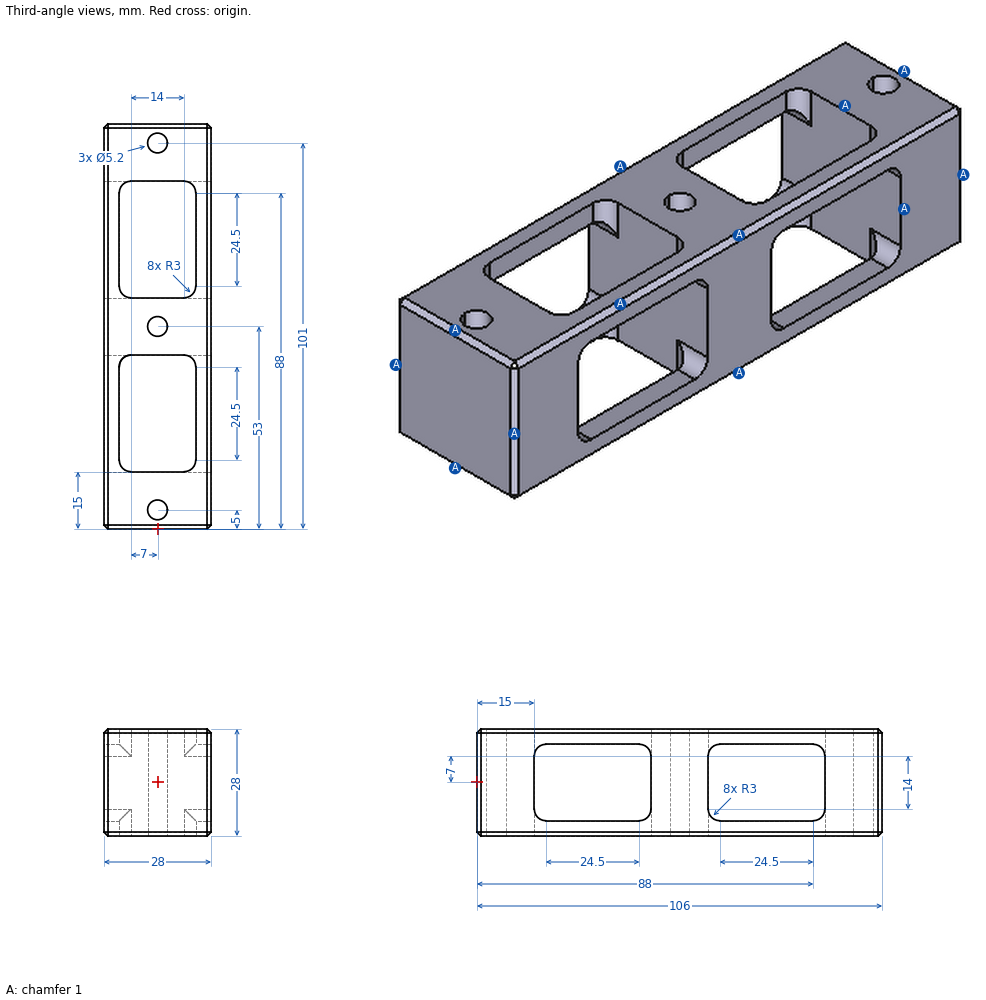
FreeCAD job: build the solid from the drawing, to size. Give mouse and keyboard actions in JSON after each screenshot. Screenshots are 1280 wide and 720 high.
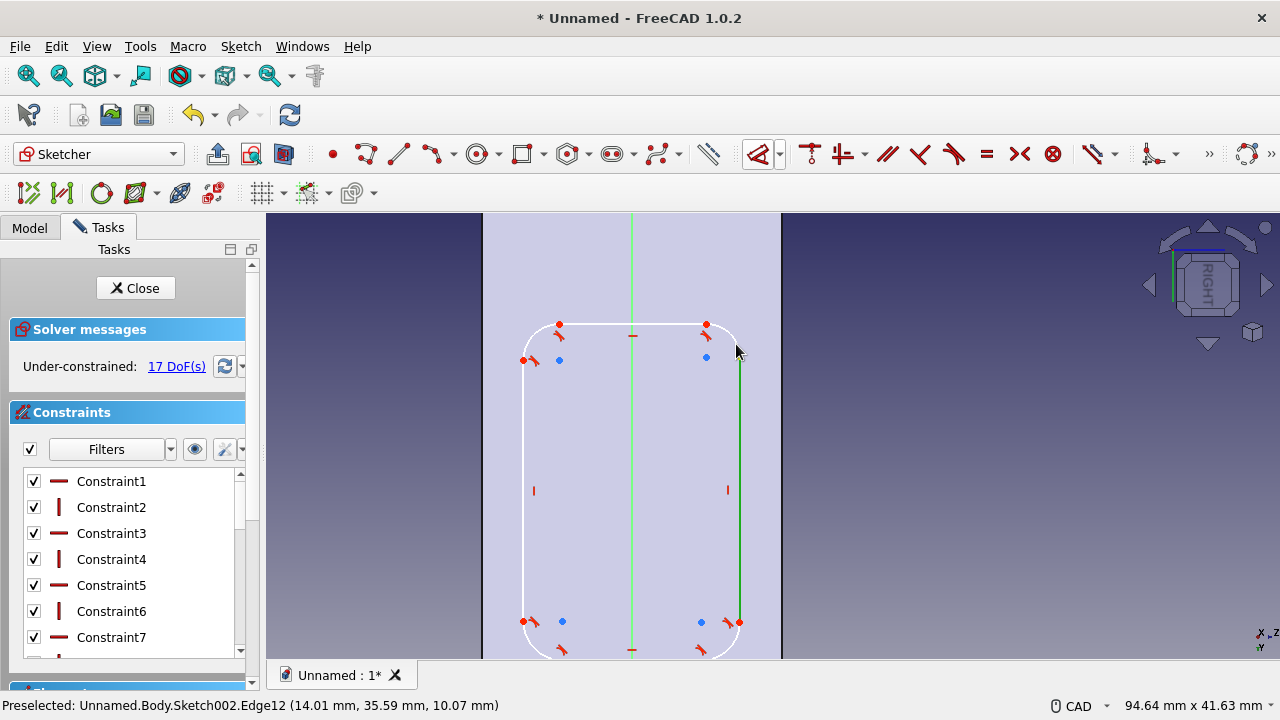
{"action": "left_click", "coordinate": [736, 342]}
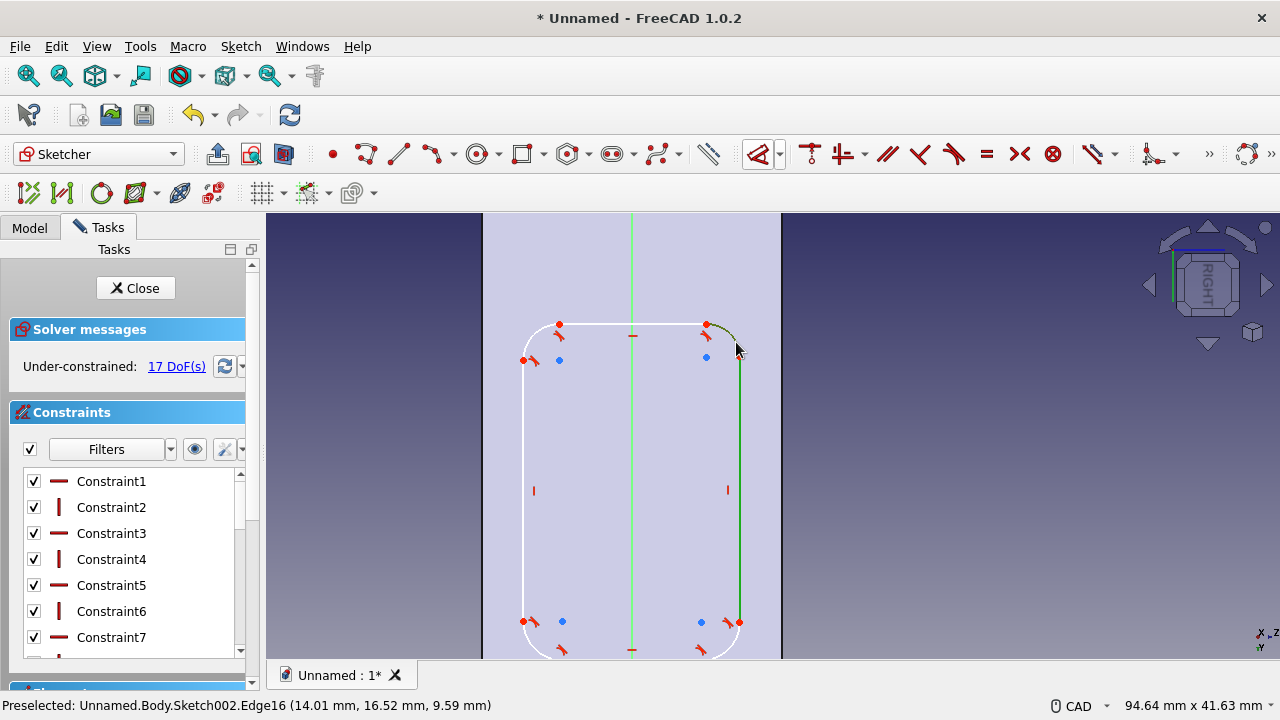
{"action": "left_click", "coordinate": [954, 154]}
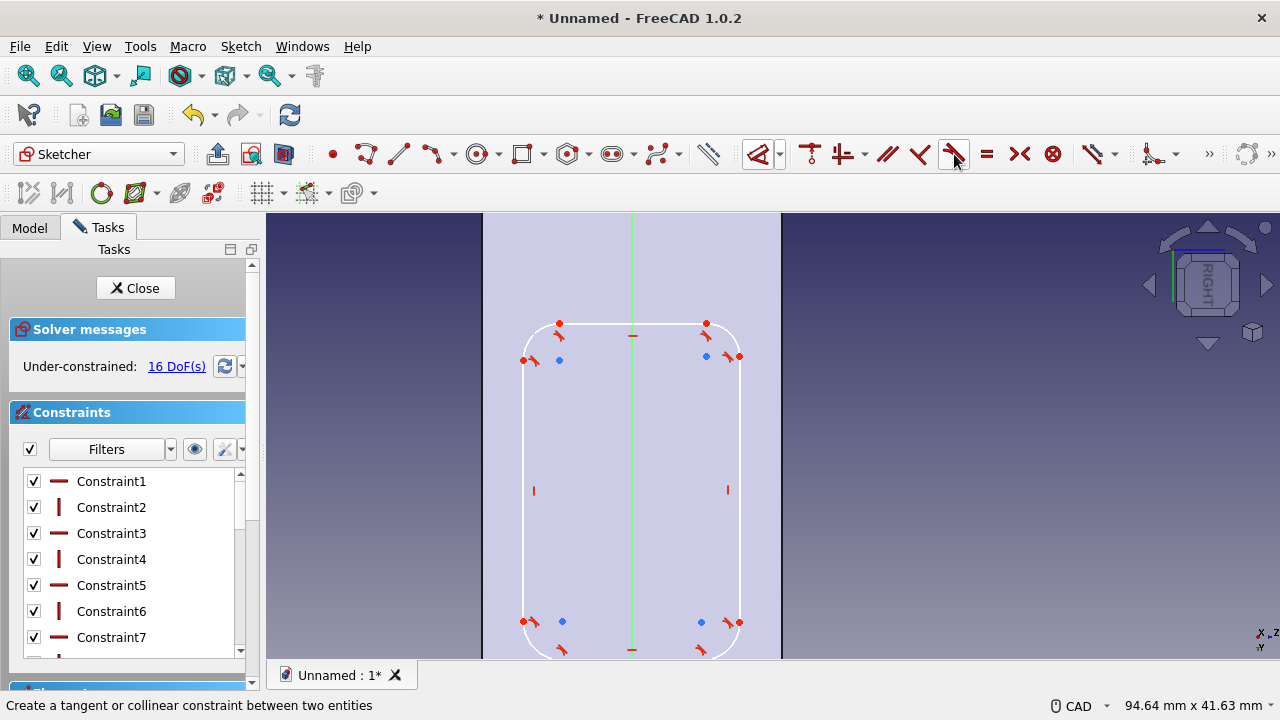
{"action": "scroll", "coordinate": [736, 344], "scroll_direction": "down", "scroll_amount": 6}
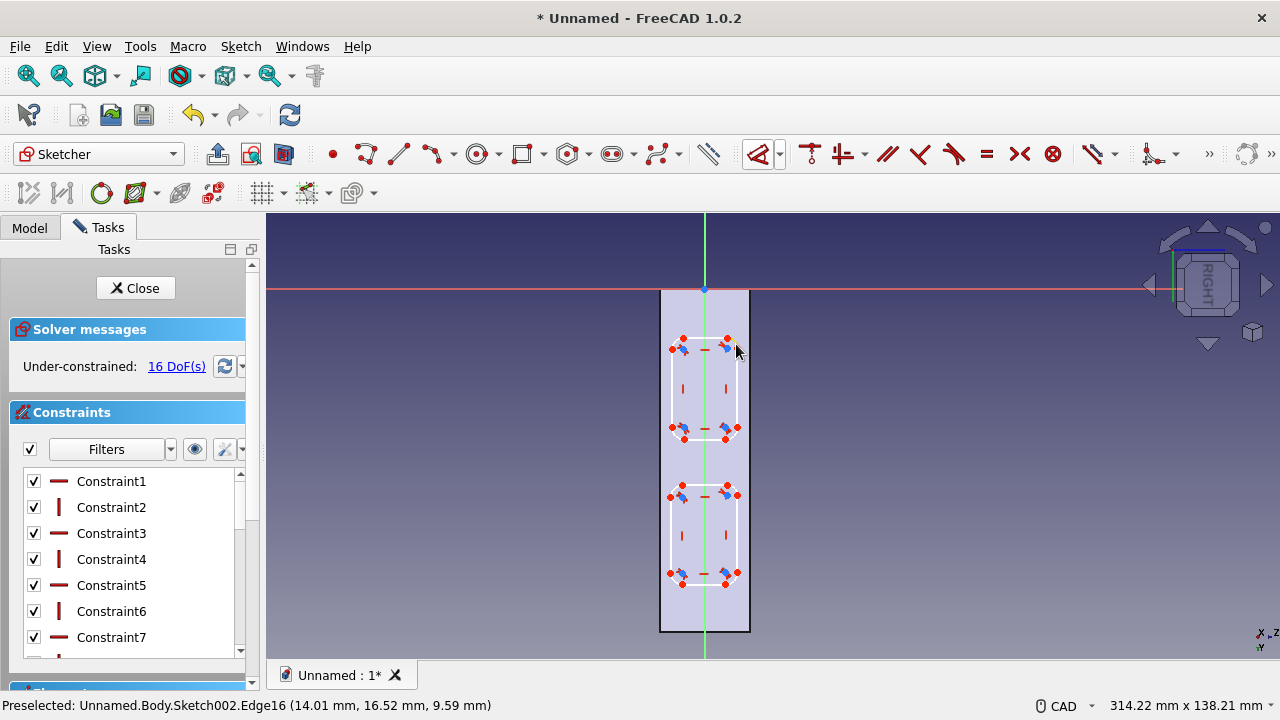
{"action": "scroll", "coordinate": [677, 487], "scroll_direction": "up", "scroll_amount": 5}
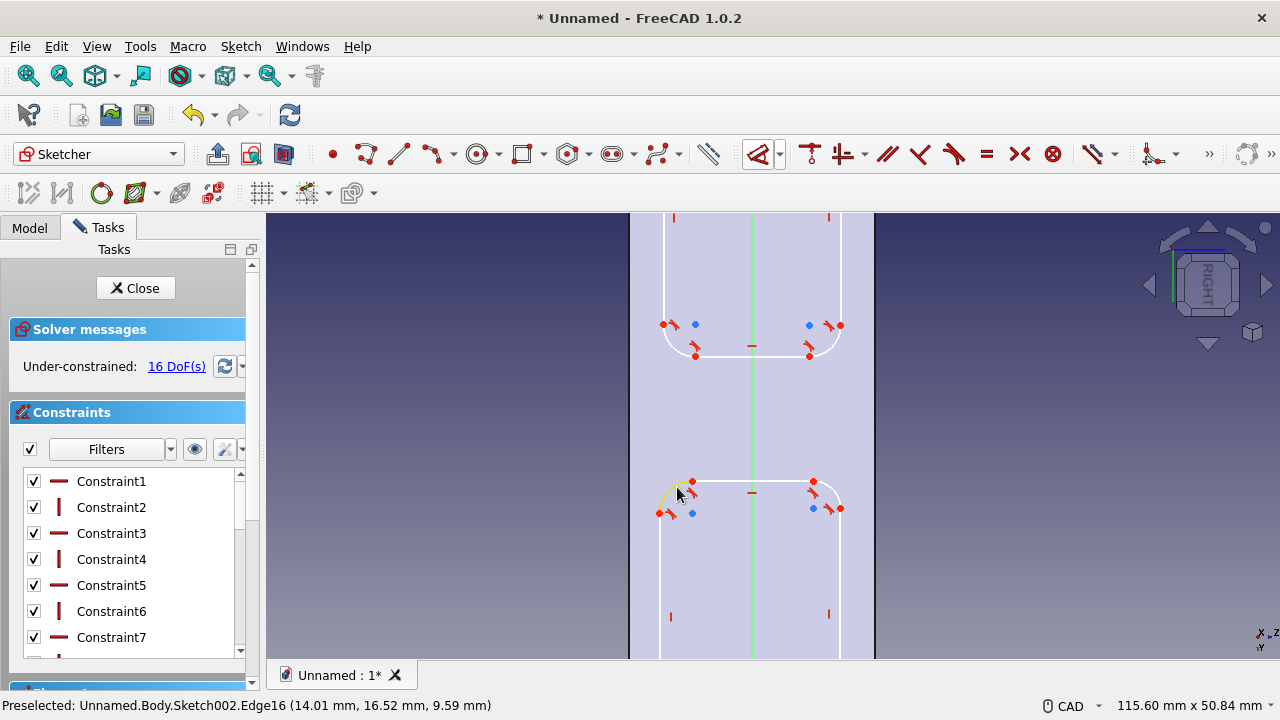
{"action": "left_click", "coordinate": [678, 485]}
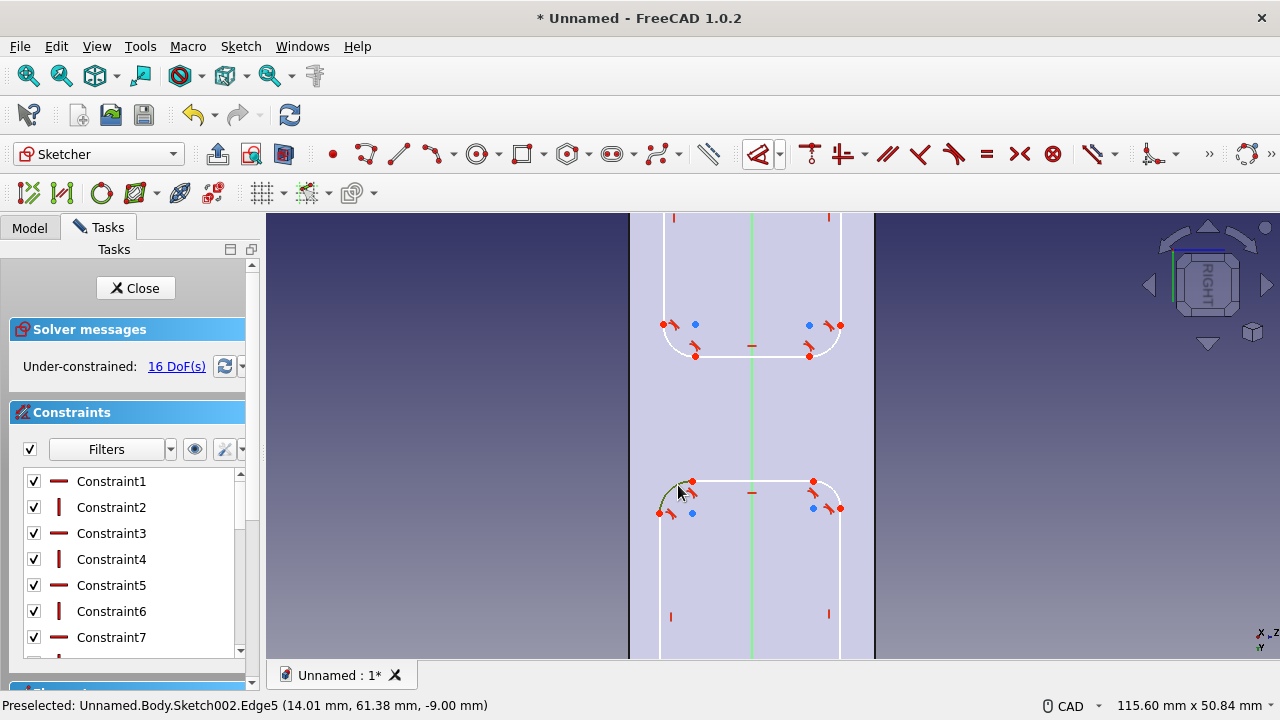
{"action": "scroll", "coordinate": [677, 487], "scroll_direction": "down", "scroll_amount": 5}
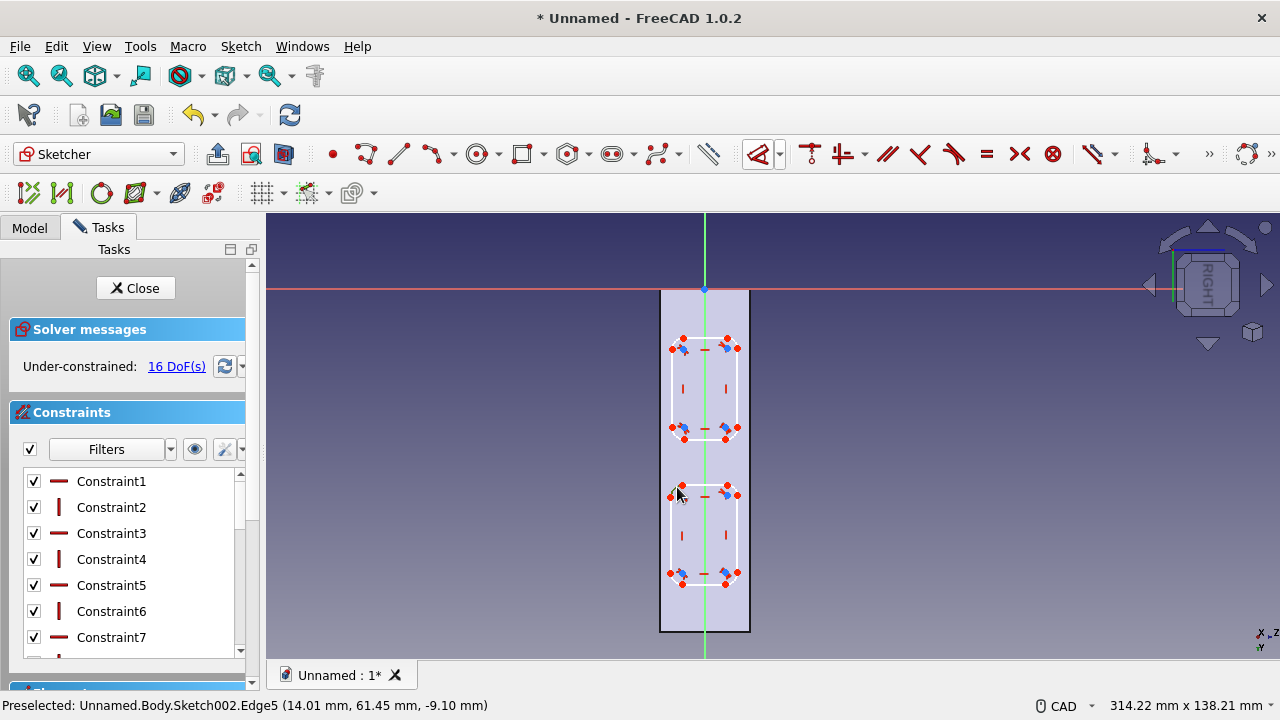
{"action": "scroll", "coordinate": [672, 578], "scroll_direction": "up", "scroll_amount": 5}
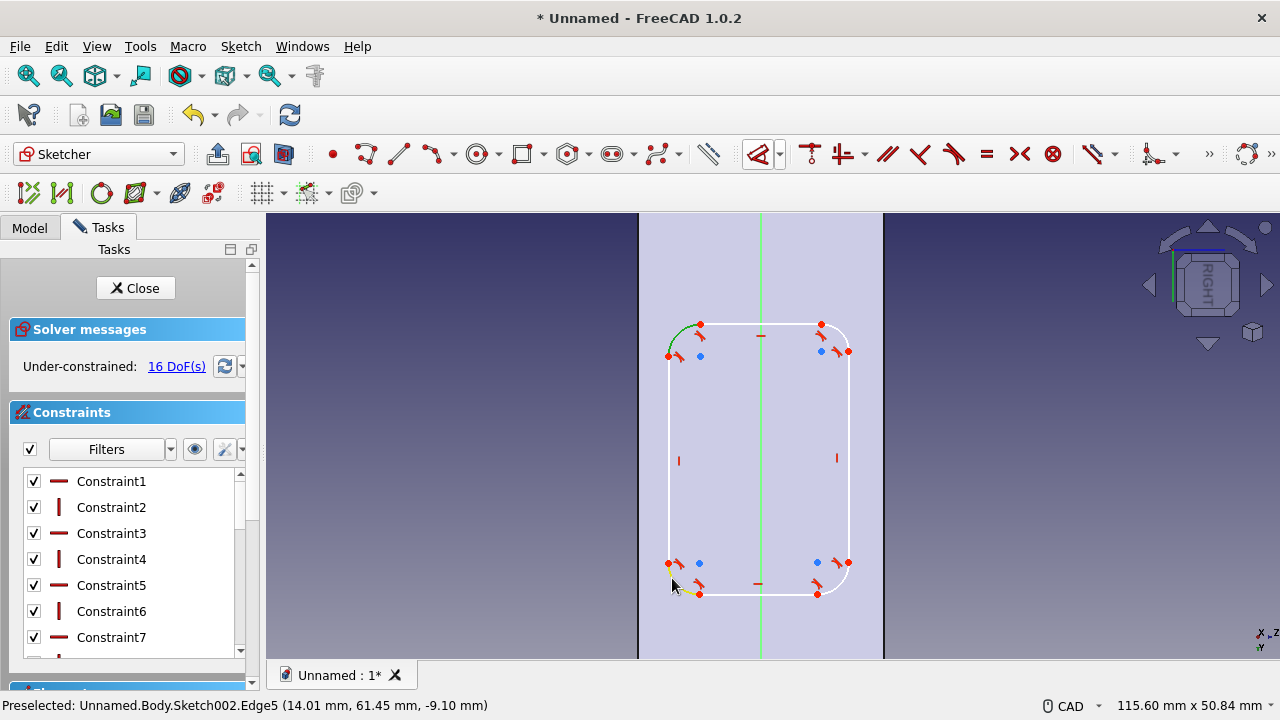
{"action": "left_click", "coordinate": [672, 577]}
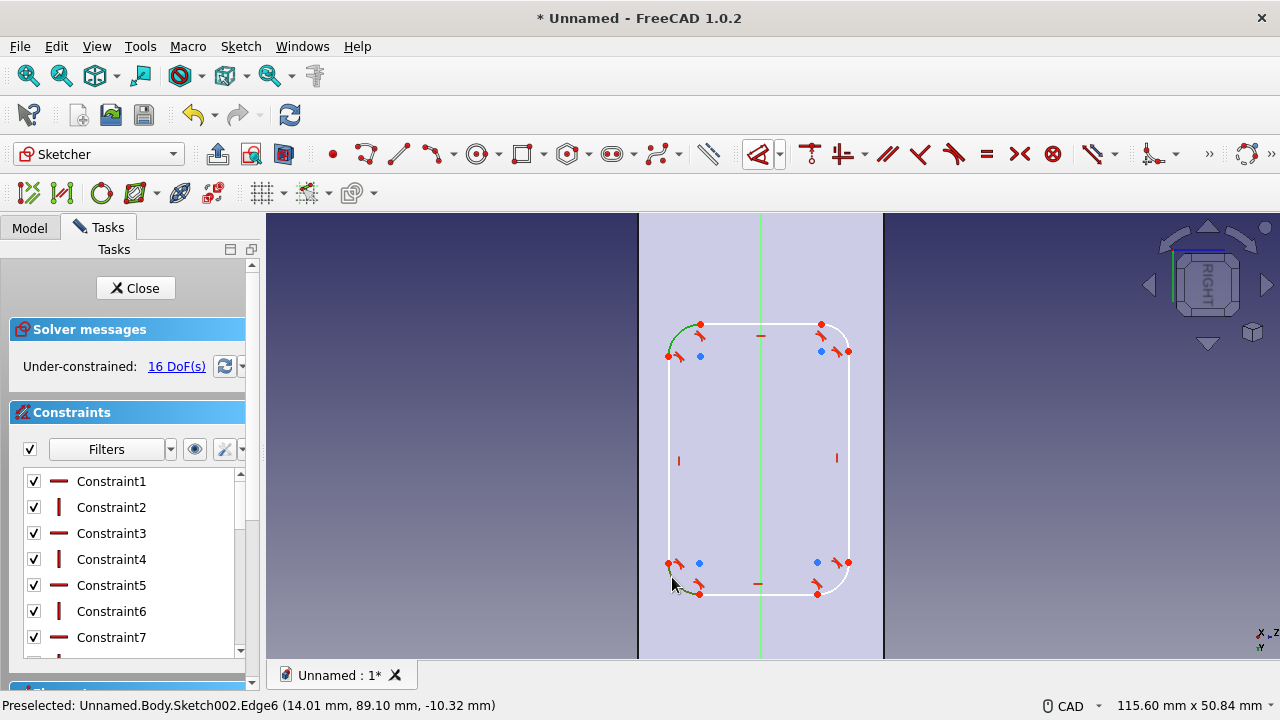
{"action": "left_click", "coordinate": [832, 591]}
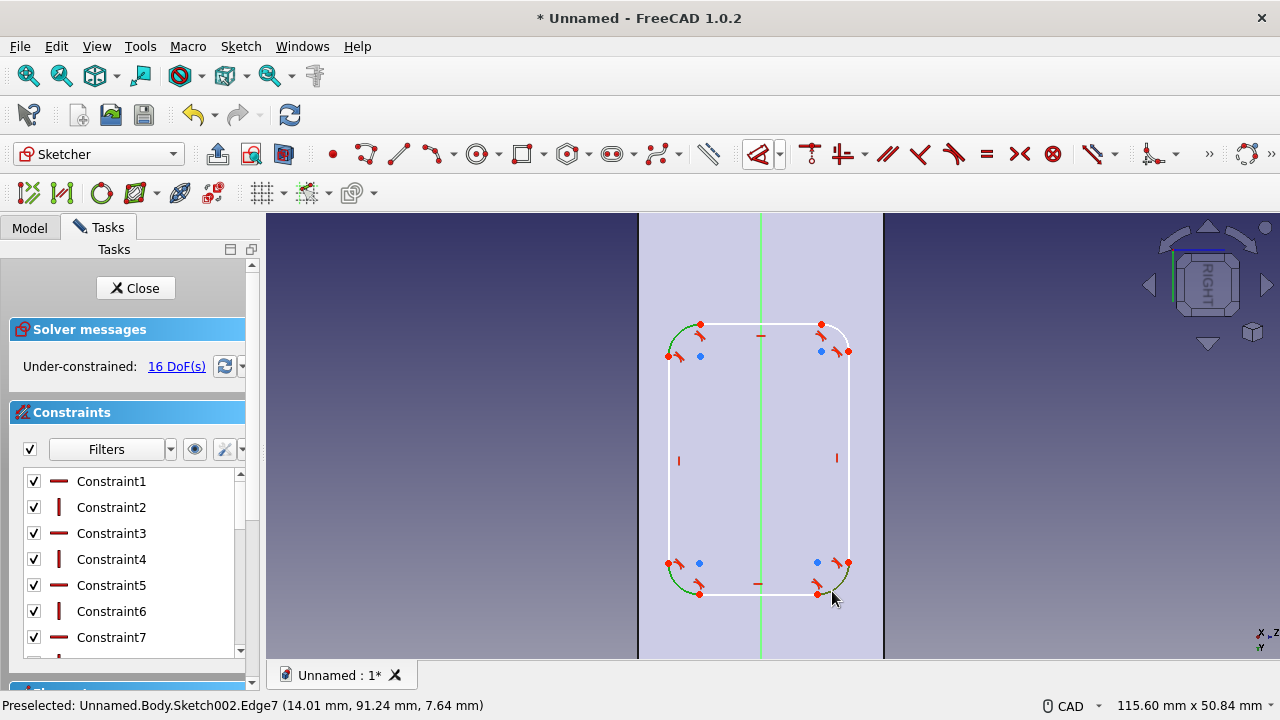
{"action": "left_click", "coordinate": [846, 339]}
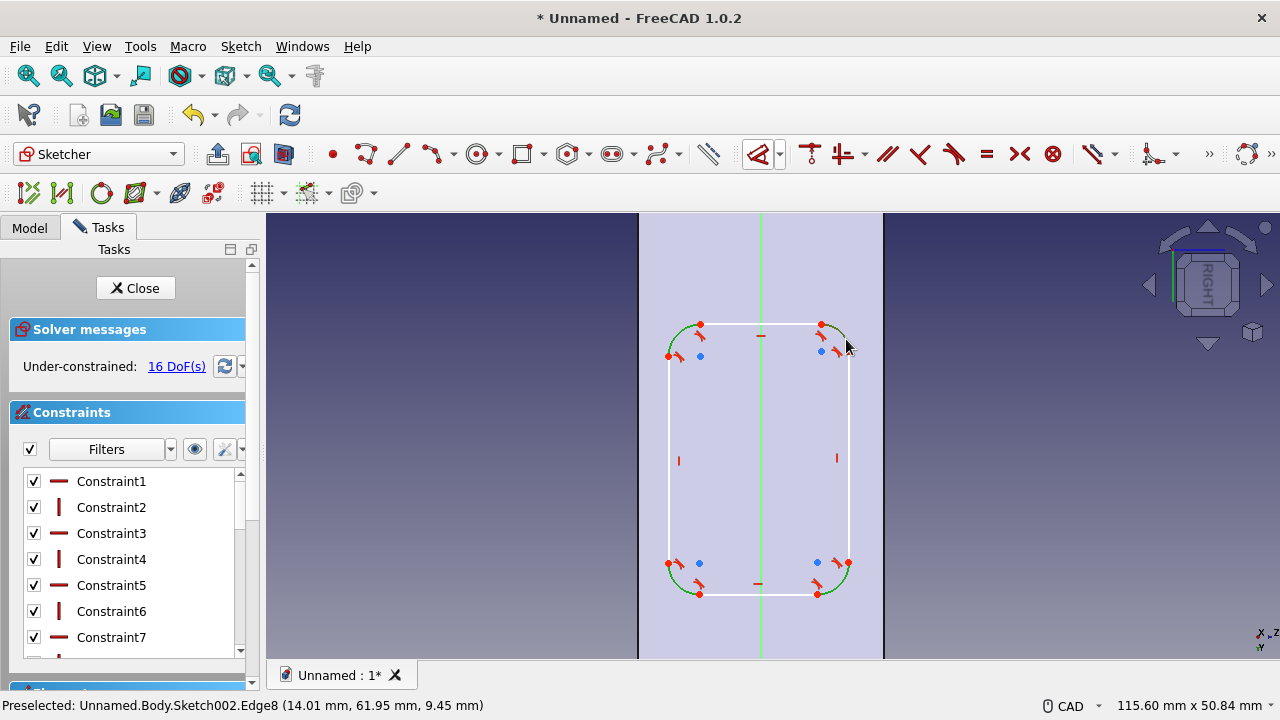
{"action": "scroll", "coordinate": [672, 578], "scroll_direction": "down", "scroll_amount": 5}